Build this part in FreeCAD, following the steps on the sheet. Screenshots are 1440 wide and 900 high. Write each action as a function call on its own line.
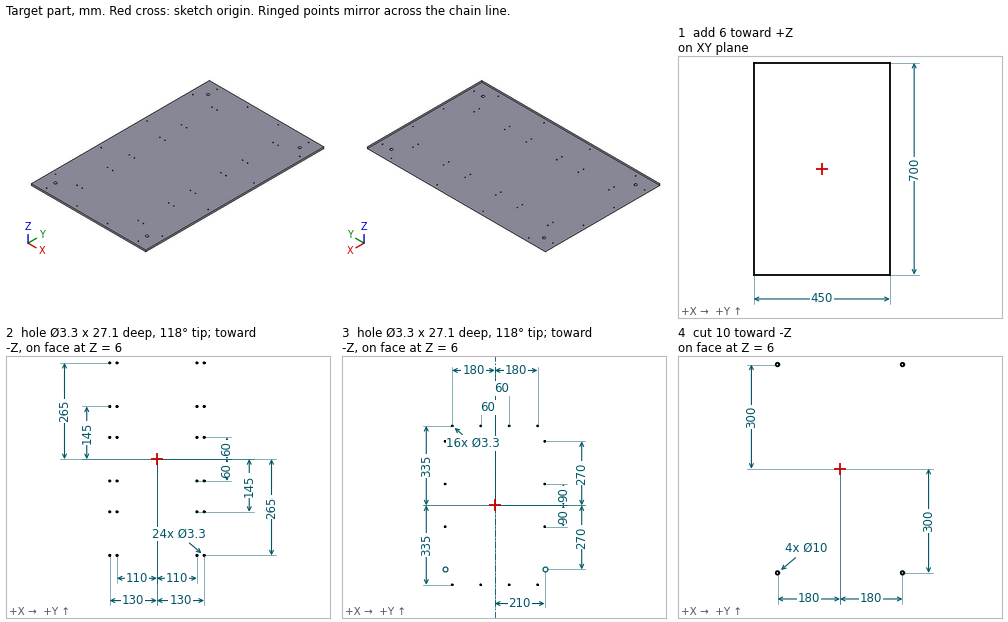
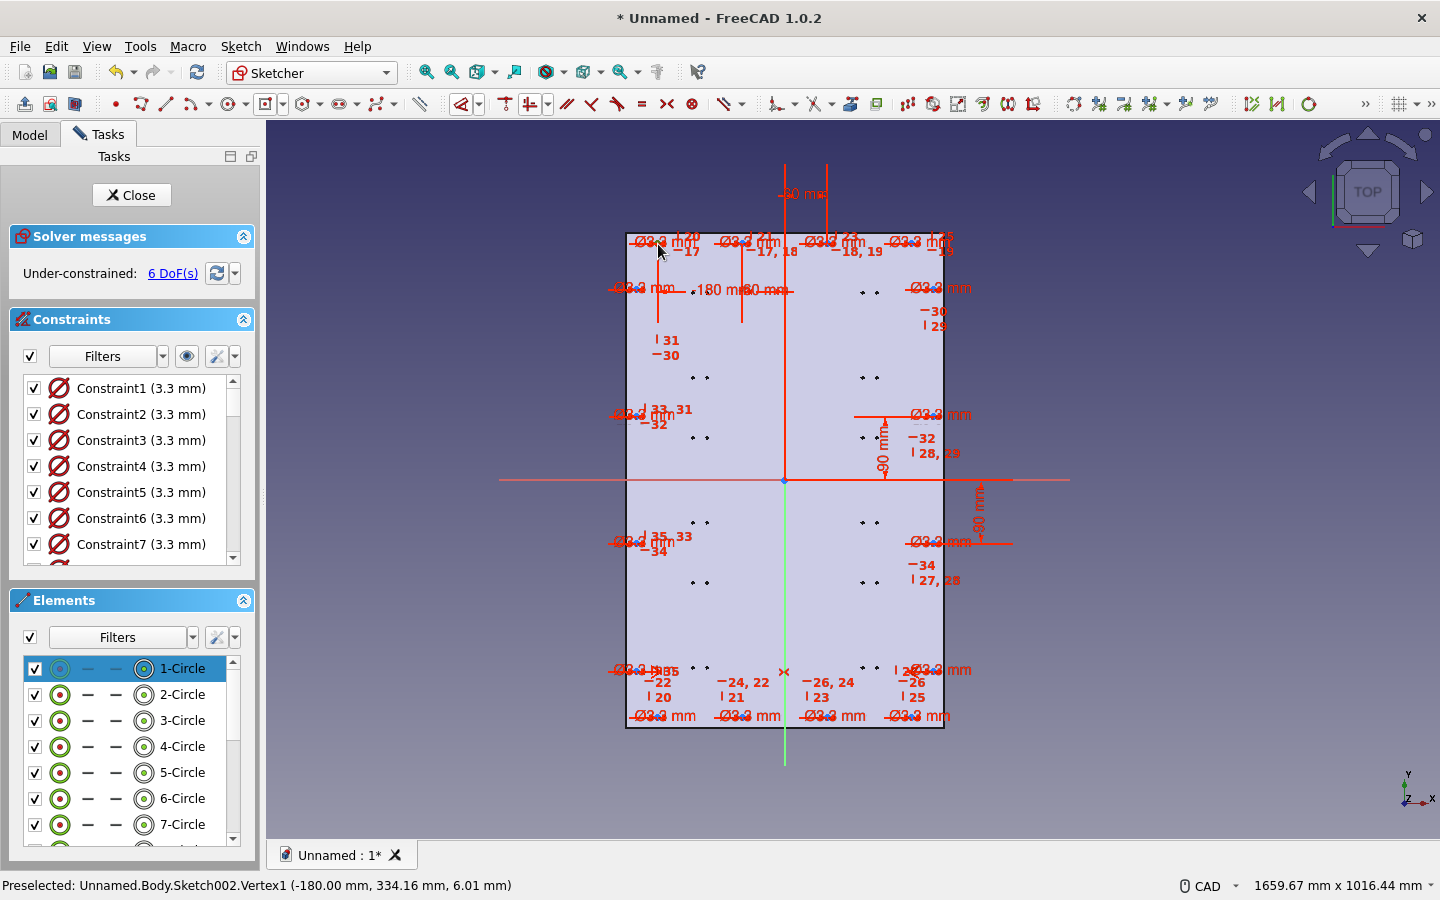
key(i)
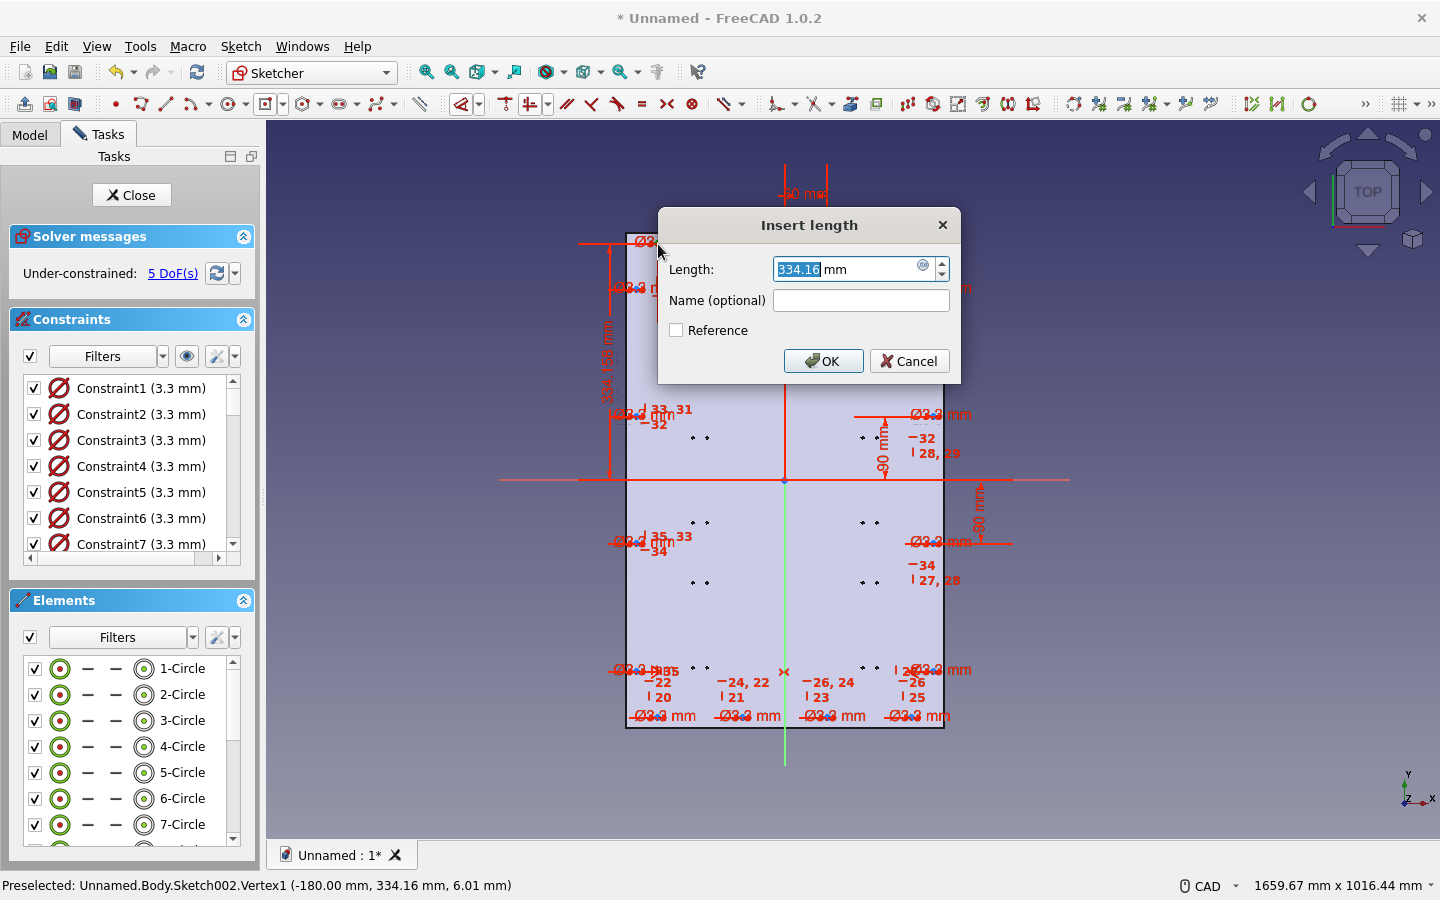
text(335)
key(Return)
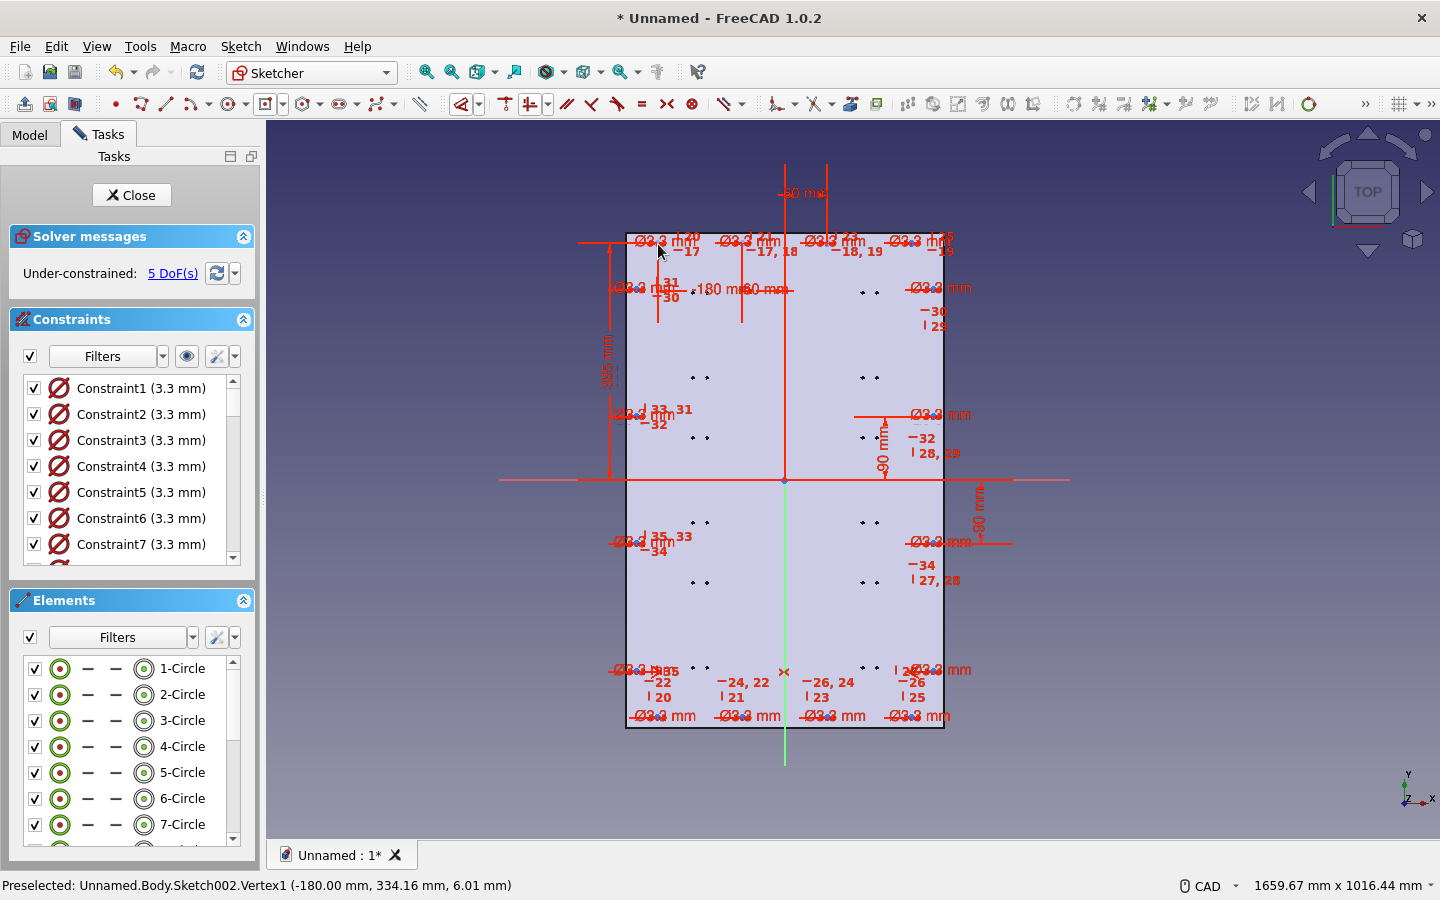
click(912, 243)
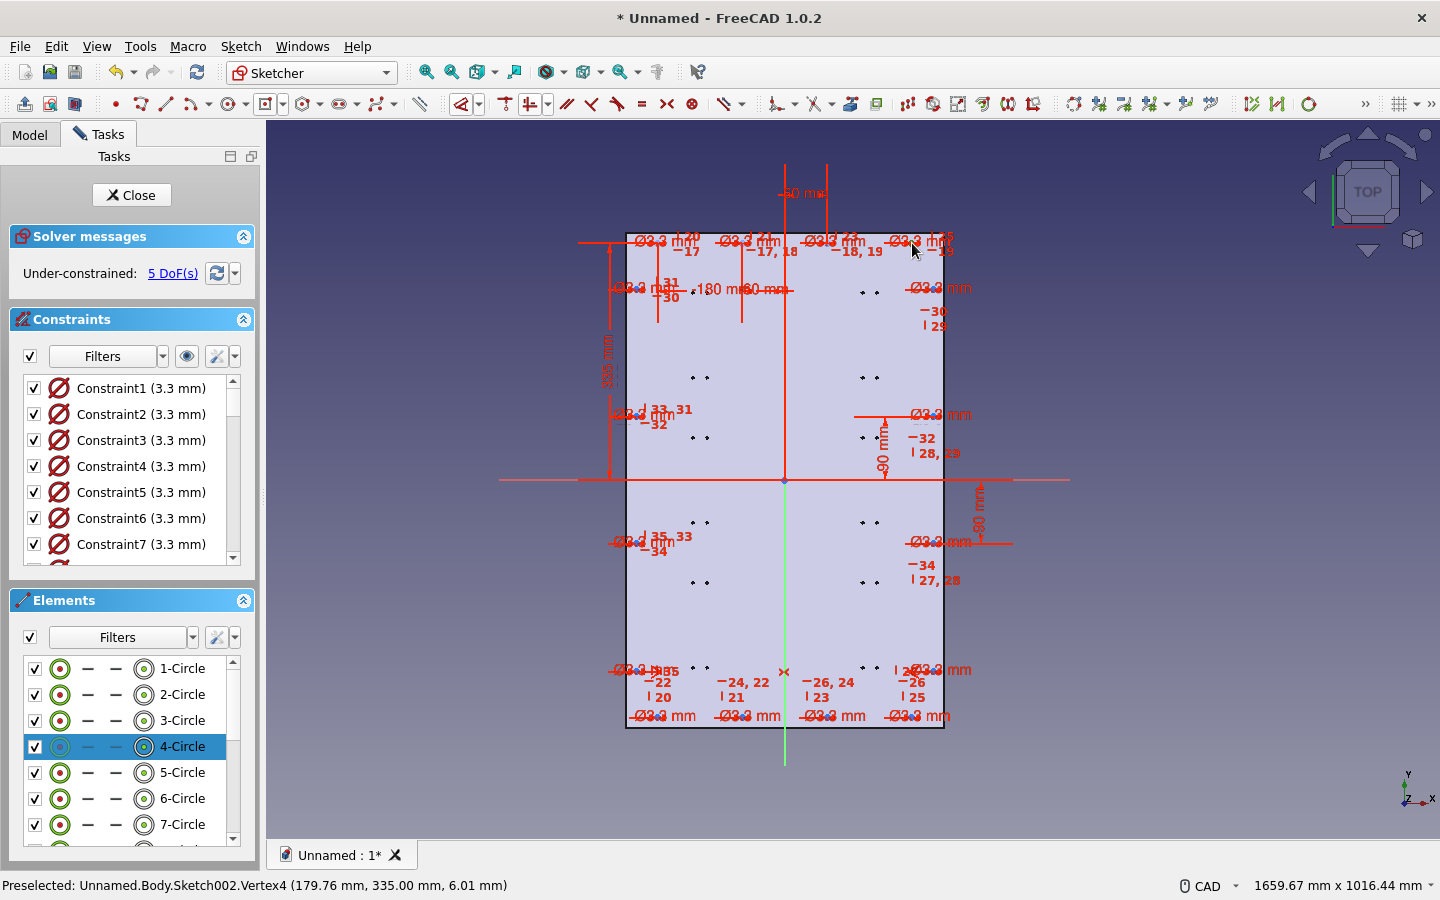
click(478, 104)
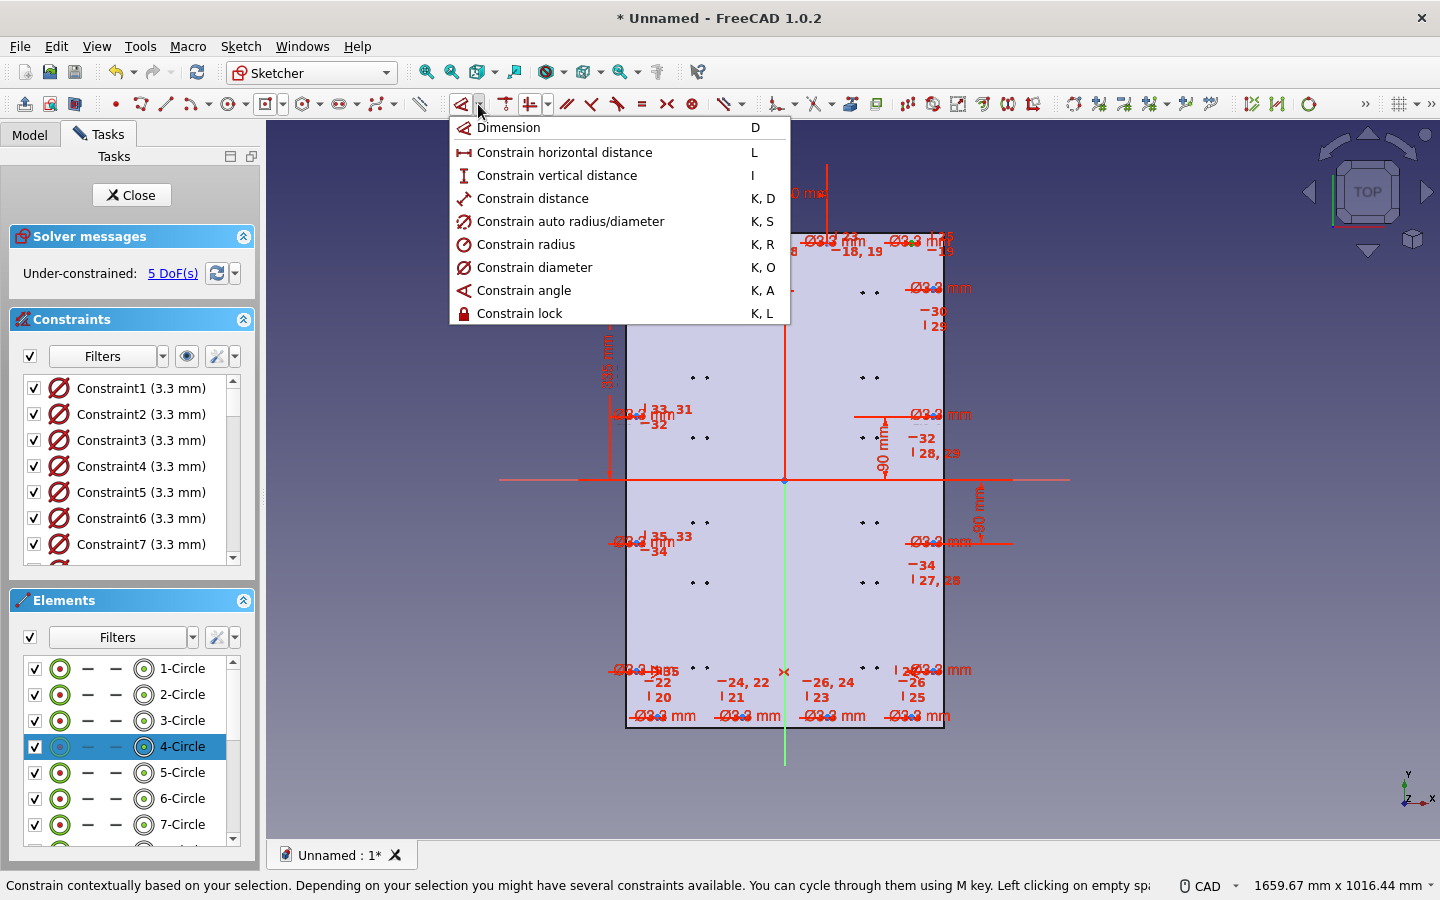
click(620, 152)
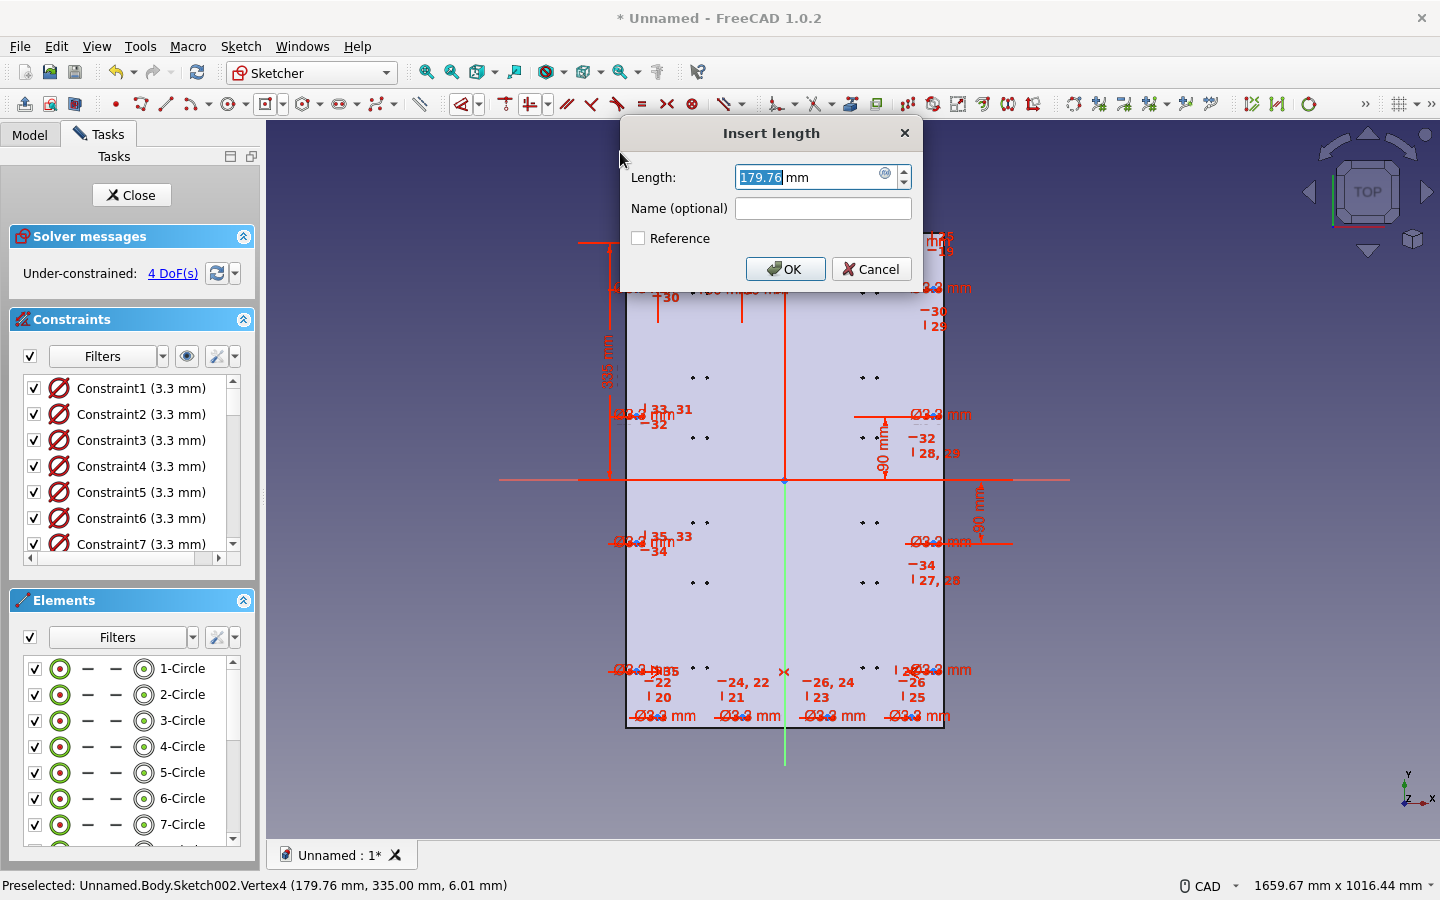
text(180)
key(Return)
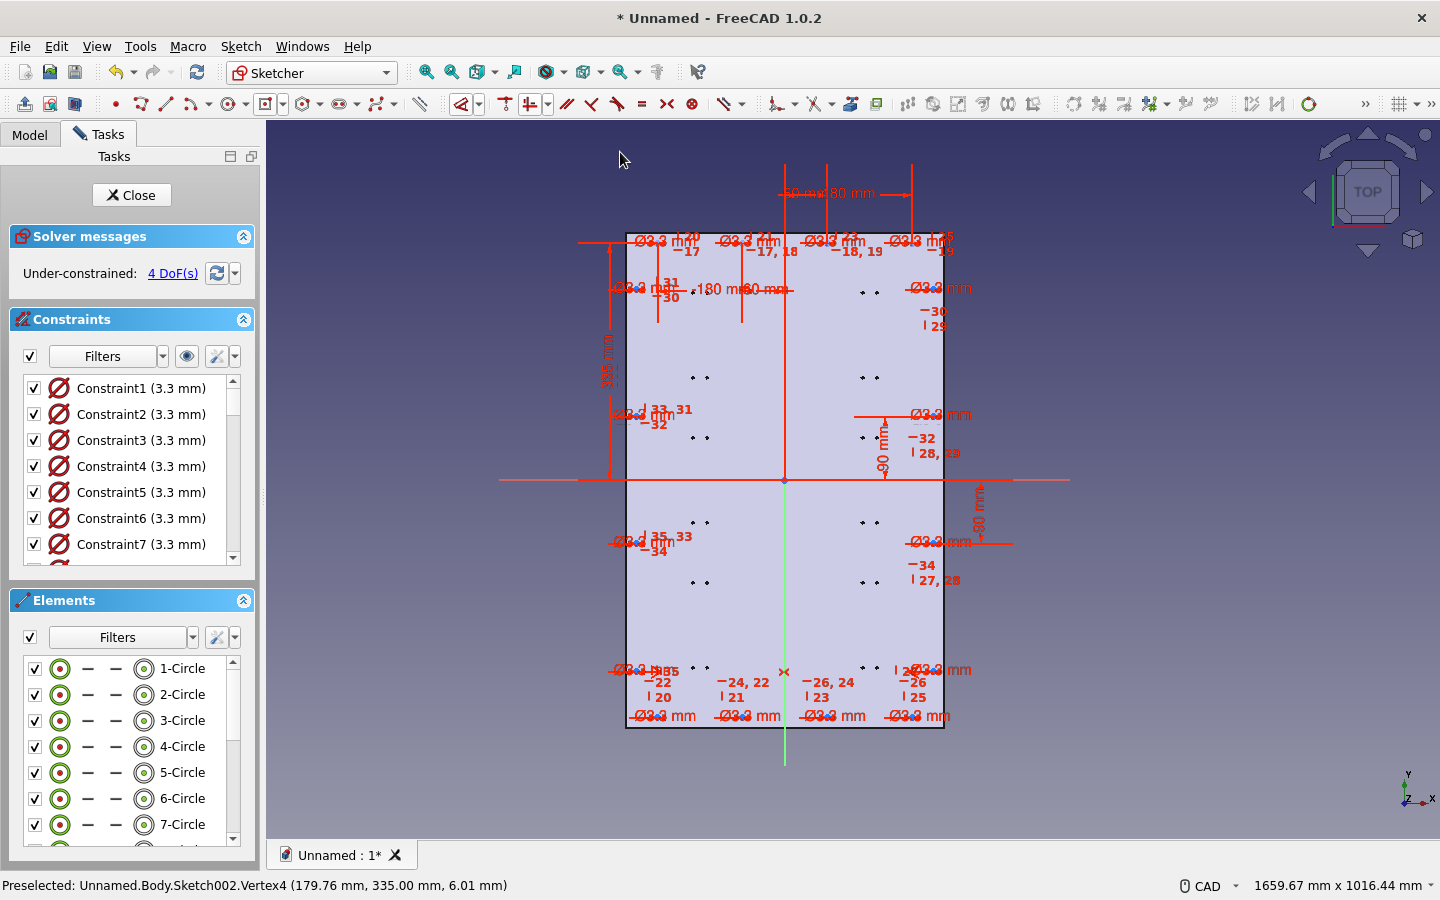
click(658, 718)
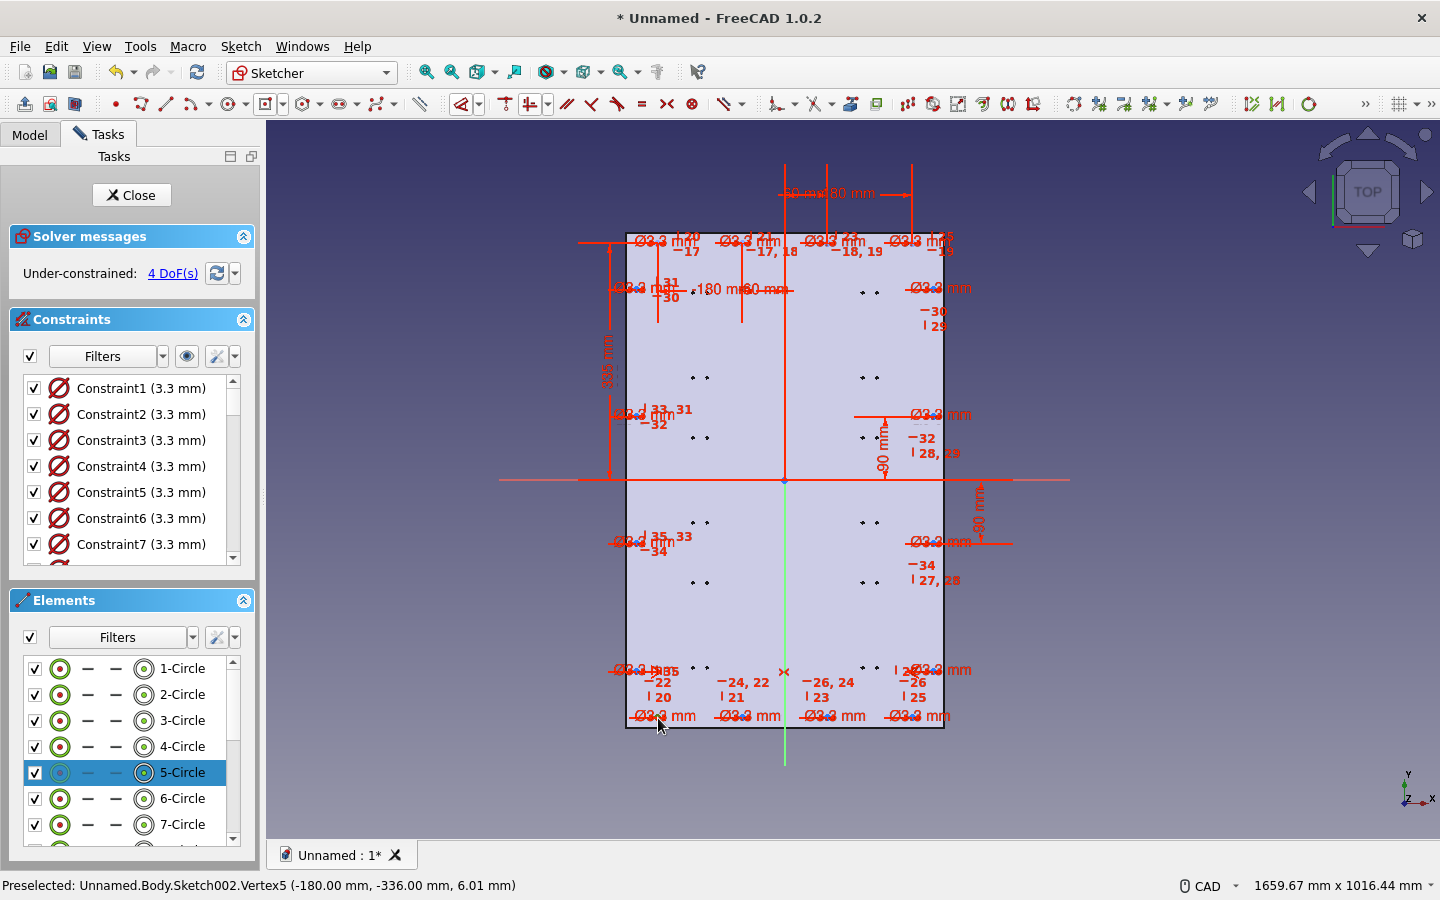
key(i)